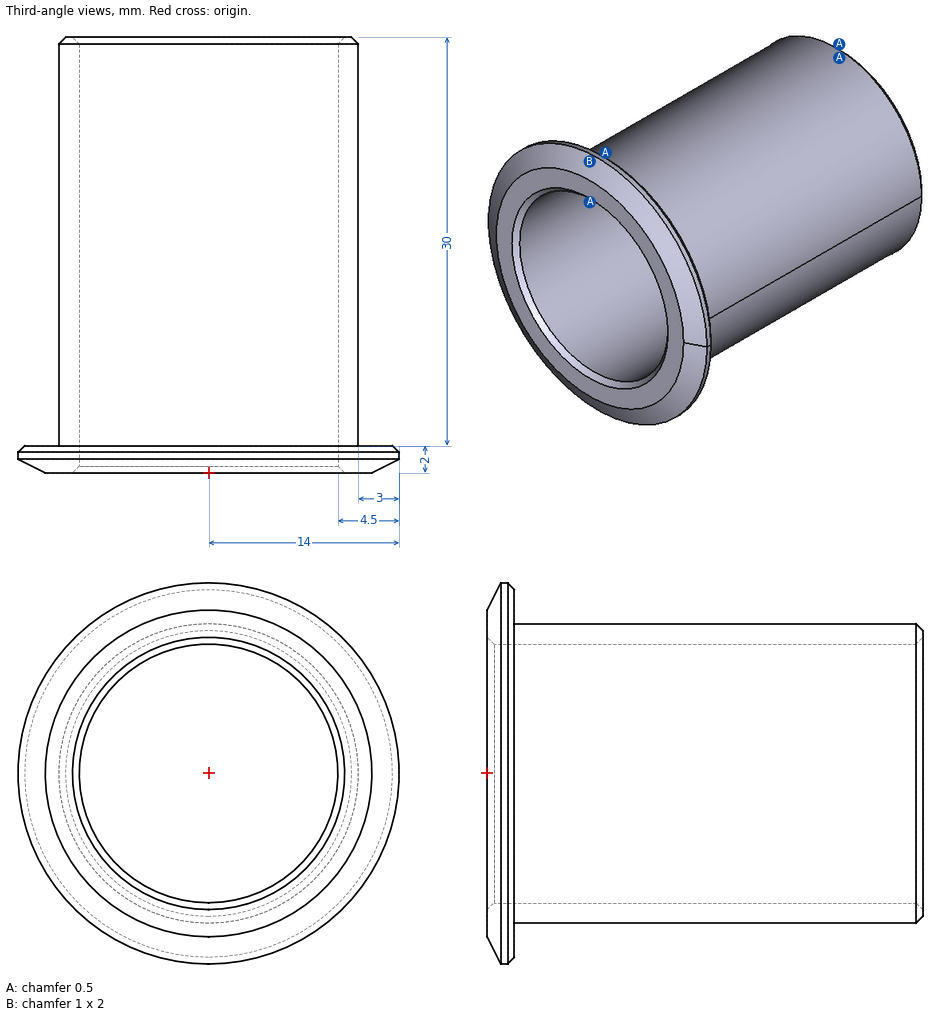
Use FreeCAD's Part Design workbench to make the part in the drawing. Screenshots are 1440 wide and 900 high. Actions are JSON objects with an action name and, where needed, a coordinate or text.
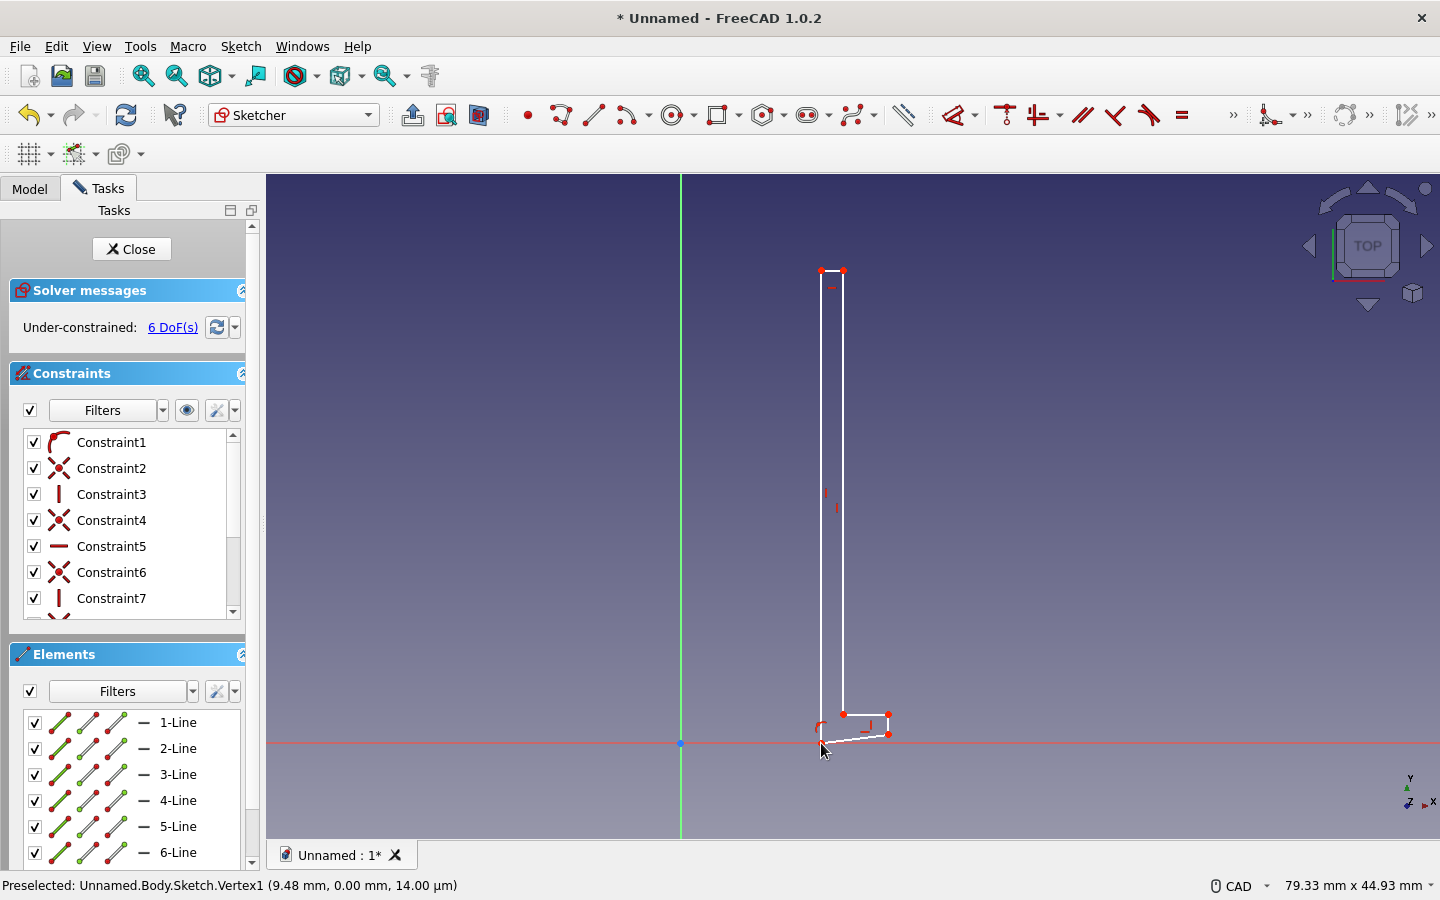
{"action": "left_click", "coordinate": [841, 741]}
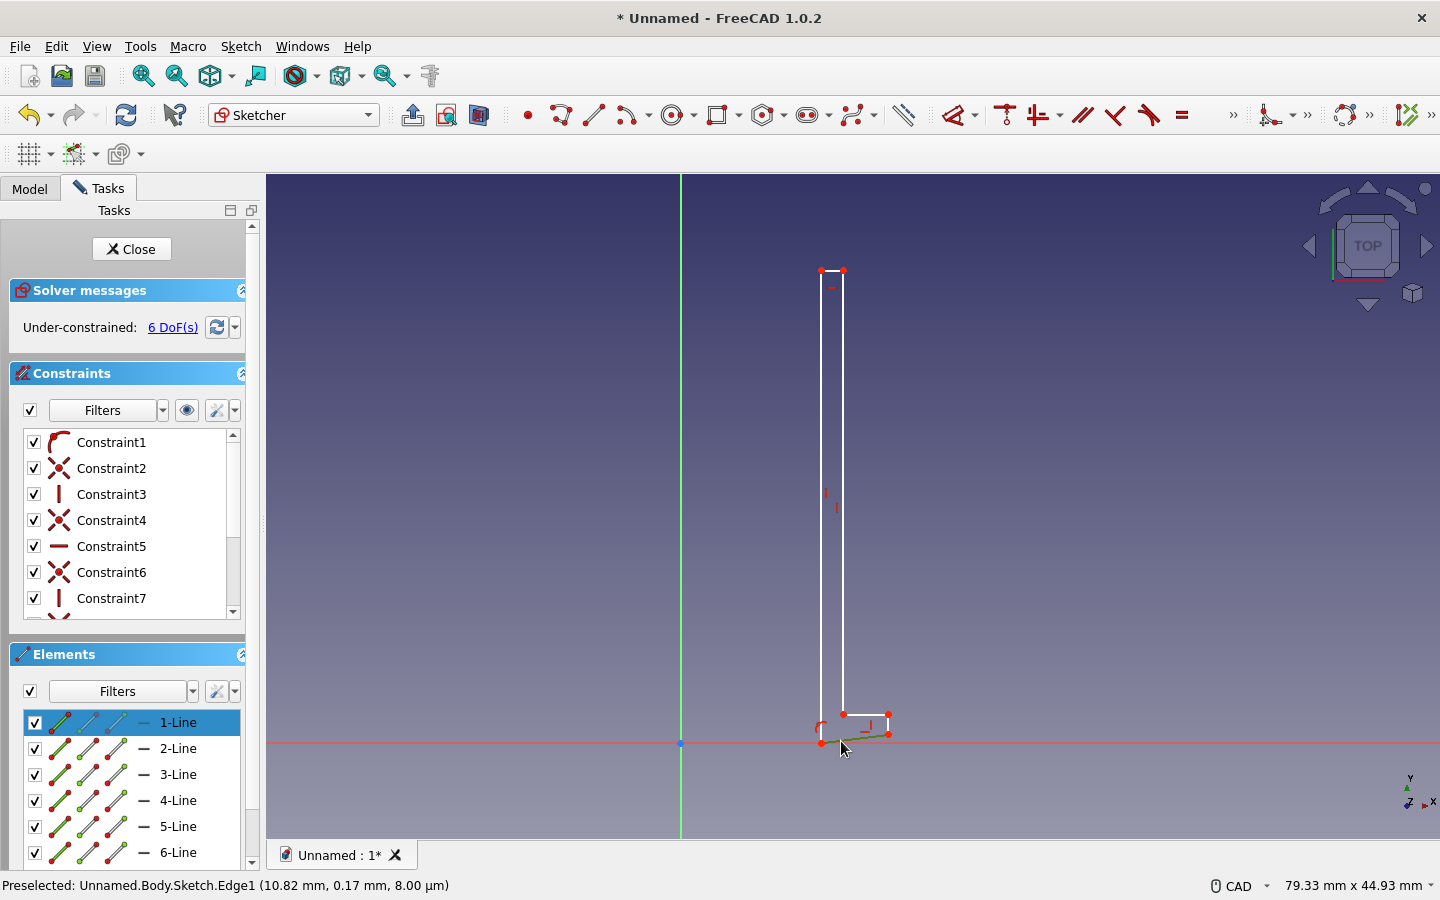
{"action": "left_click", "coordinate": [1060, 116]}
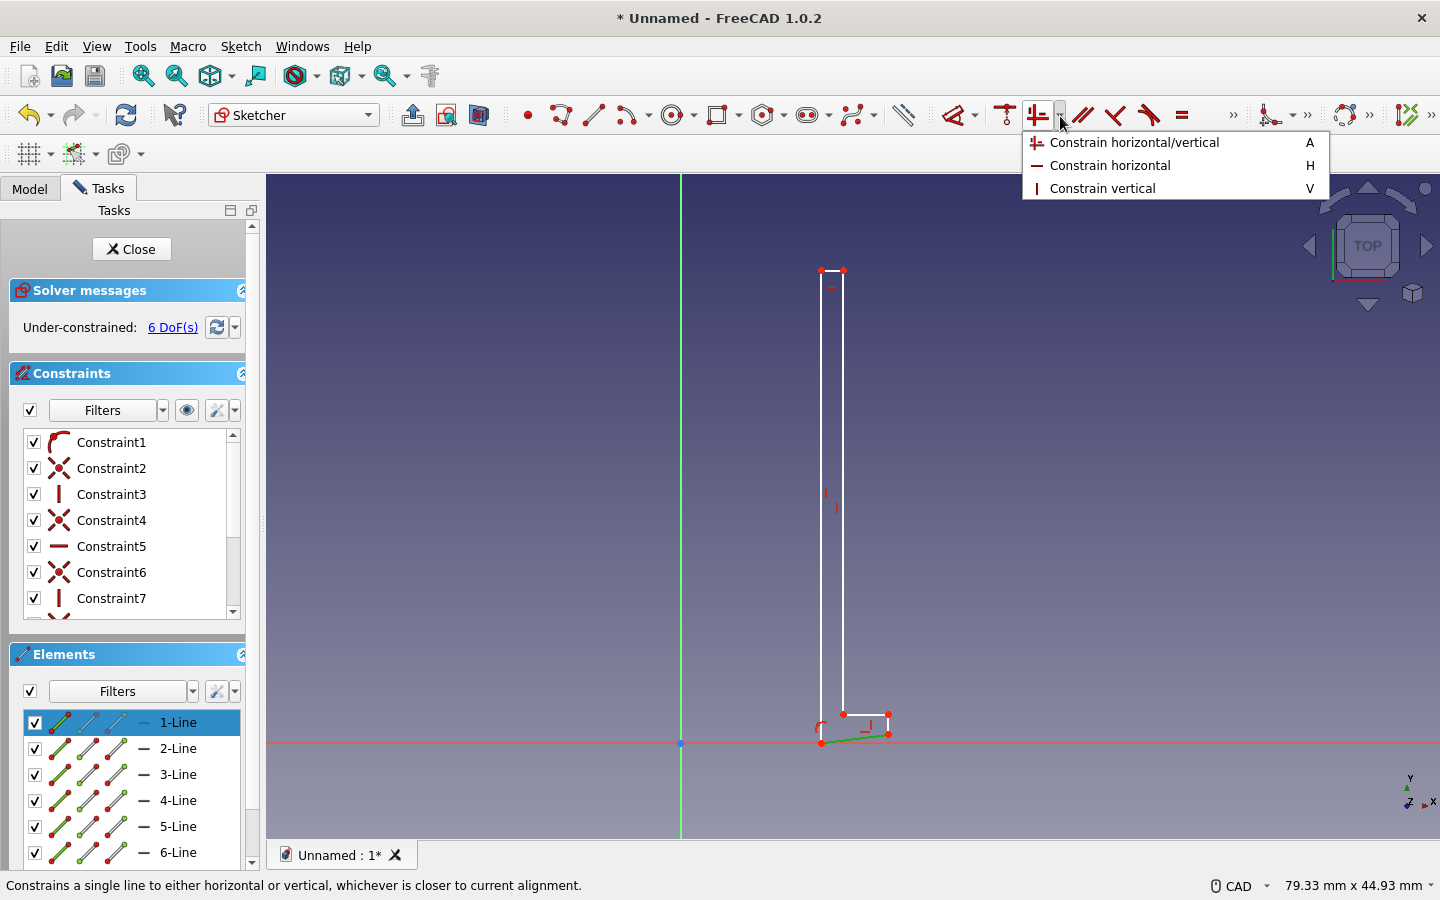
{"action": "left_click", "coordinate": [1176, 166]}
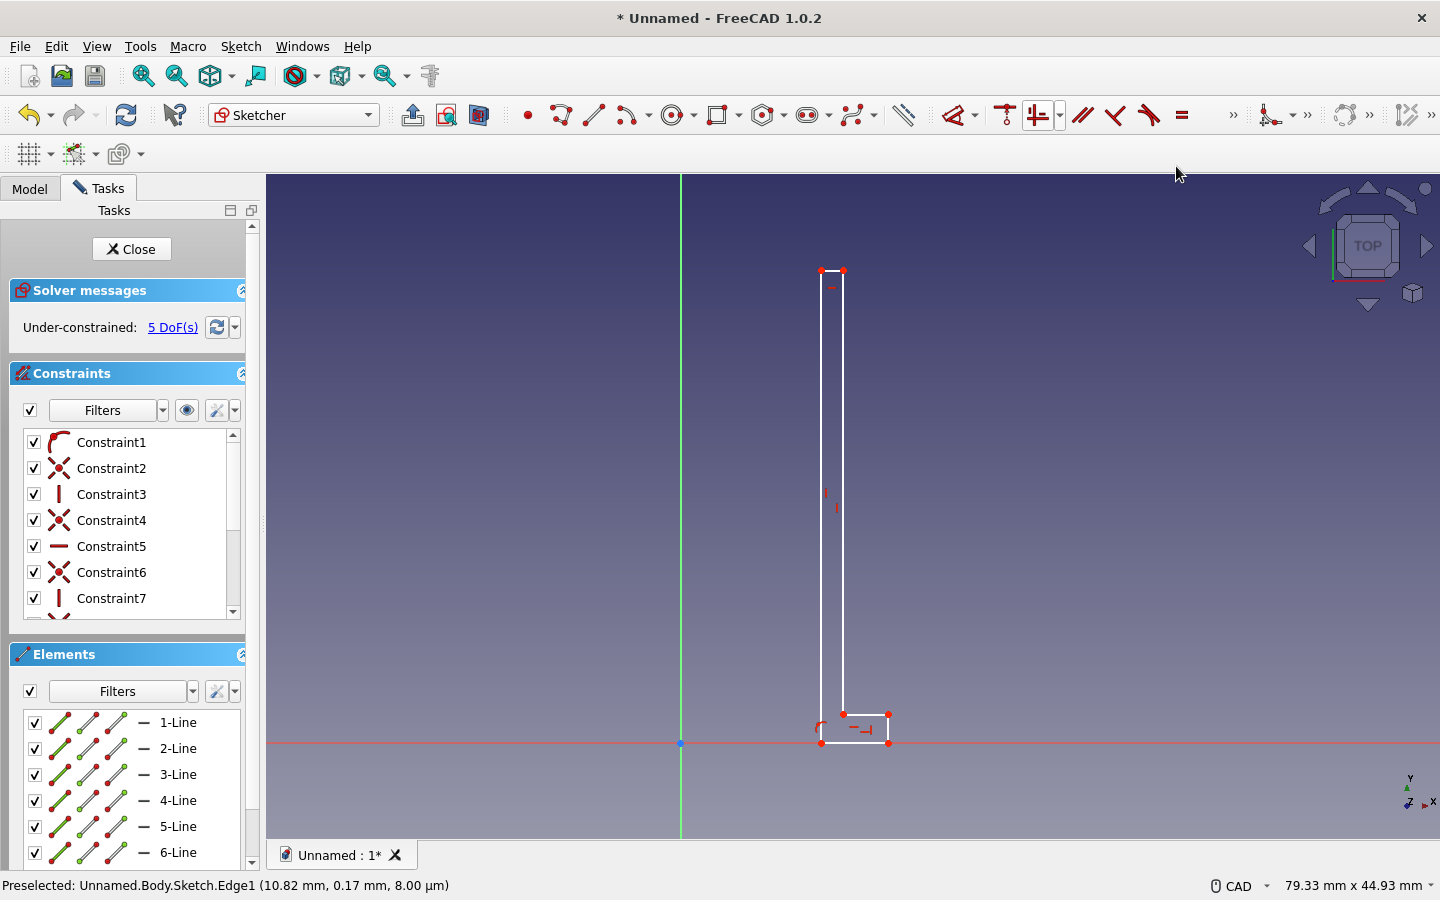
{"action": "key", "text": "d"}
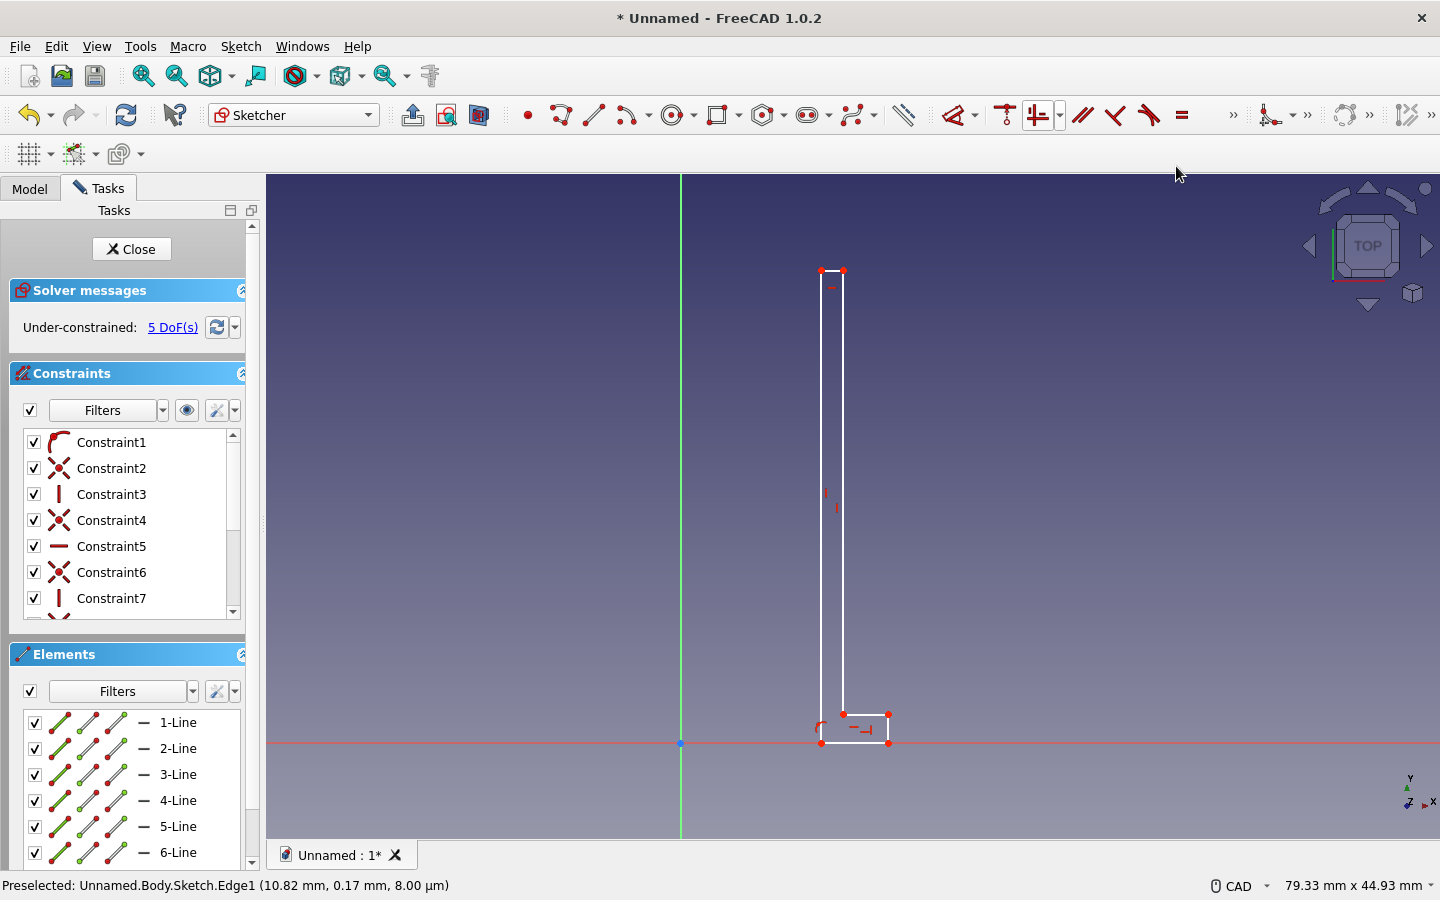
{"action": "scroll", "coordinate": [888, 732], "scroll_direction": "up", "scroll_amount": 2}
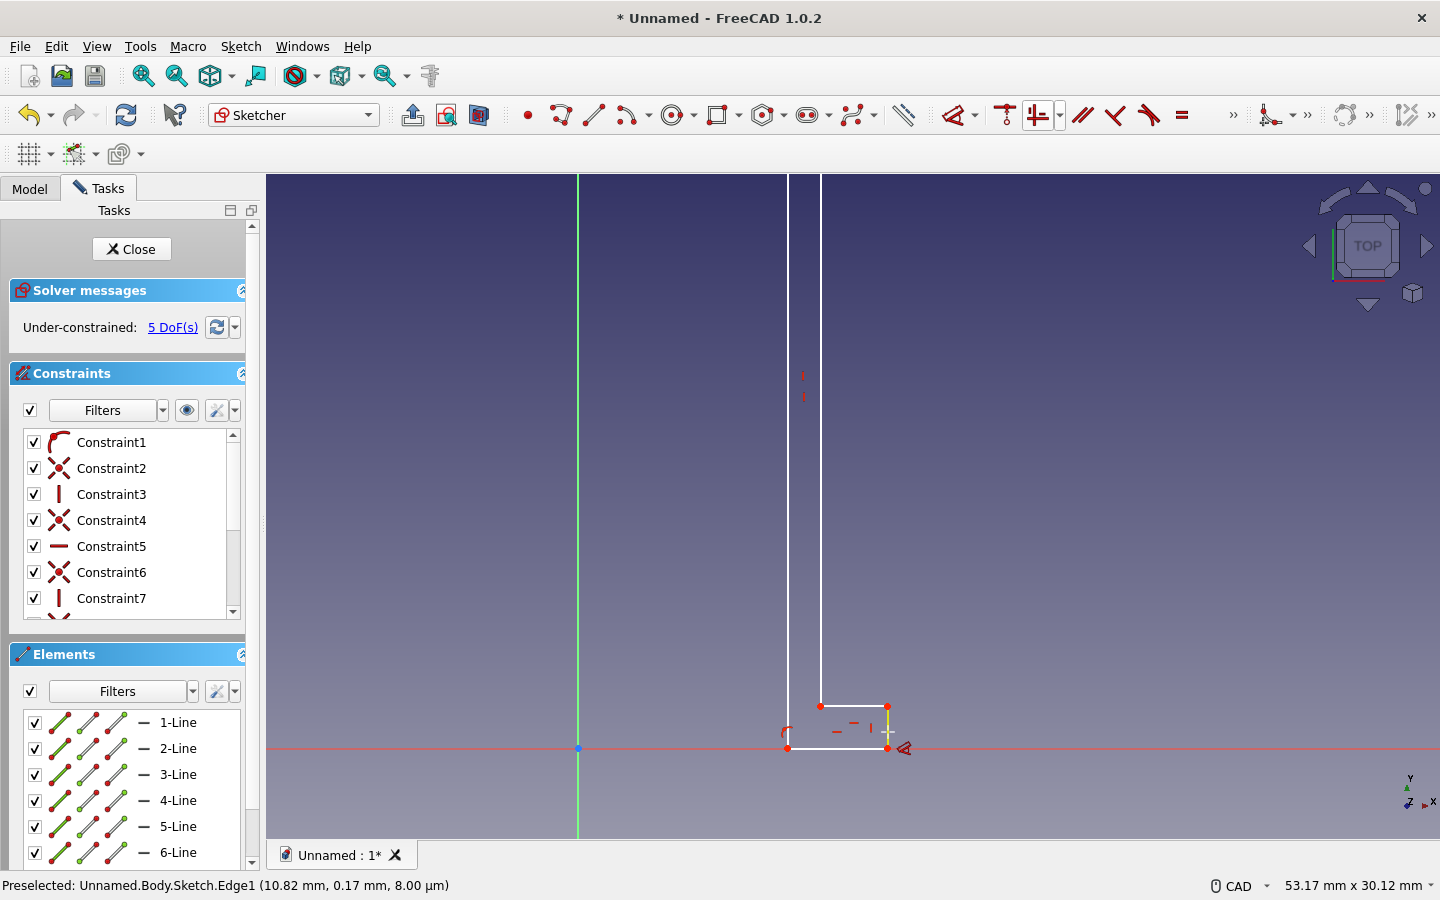
{"action": "left_click", "coordinate": [888, 732]}
{"action": "left_click", "coordinate": [922, 727]}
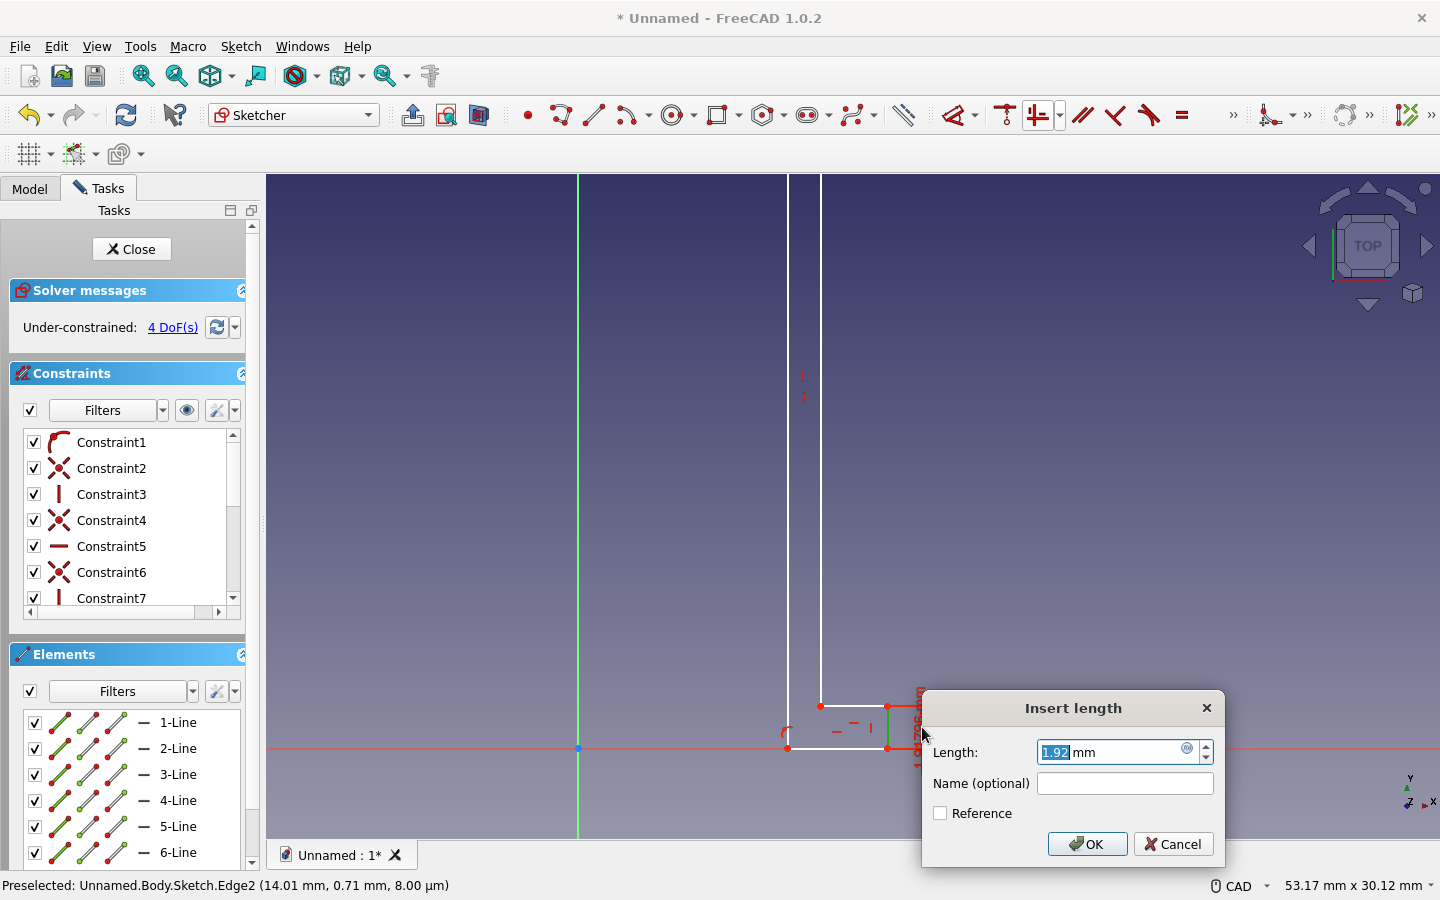
{"action": "type", "text": "2"}
{"action": "key", "text": "Return"}